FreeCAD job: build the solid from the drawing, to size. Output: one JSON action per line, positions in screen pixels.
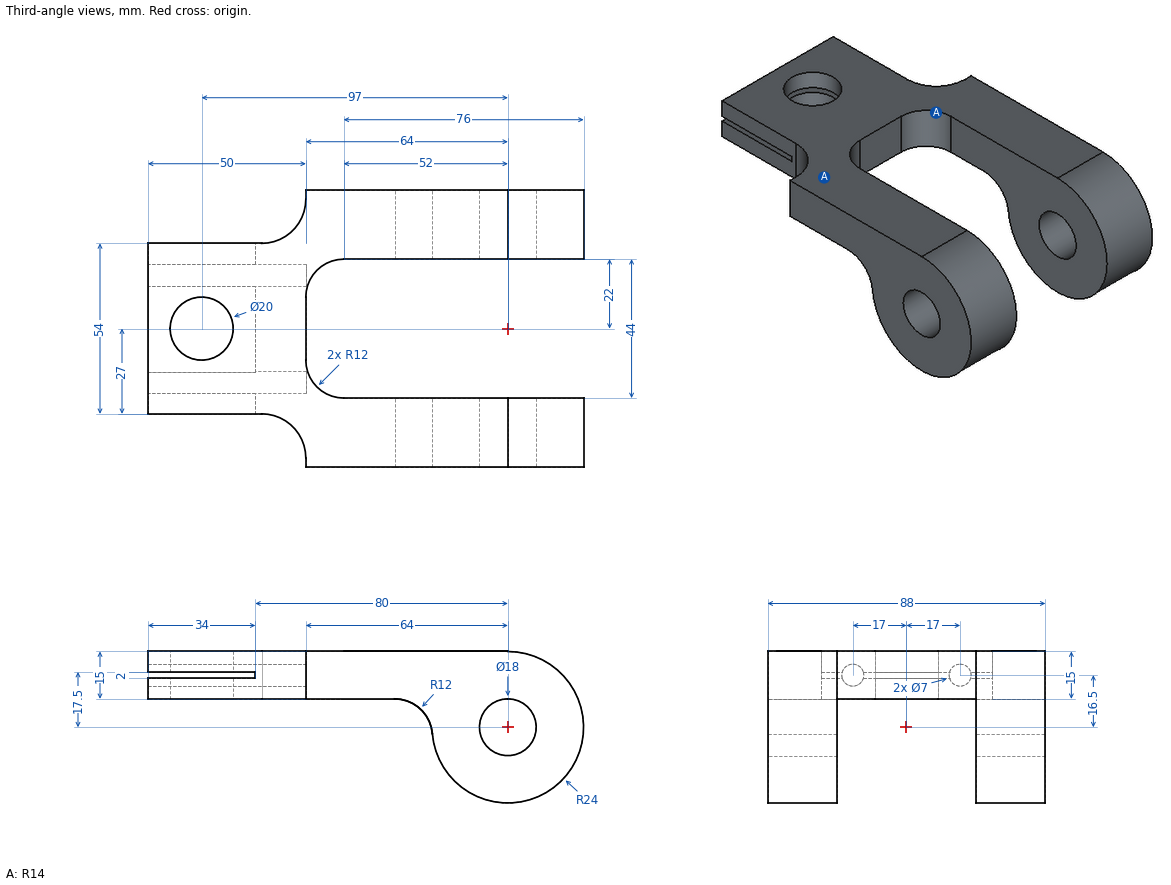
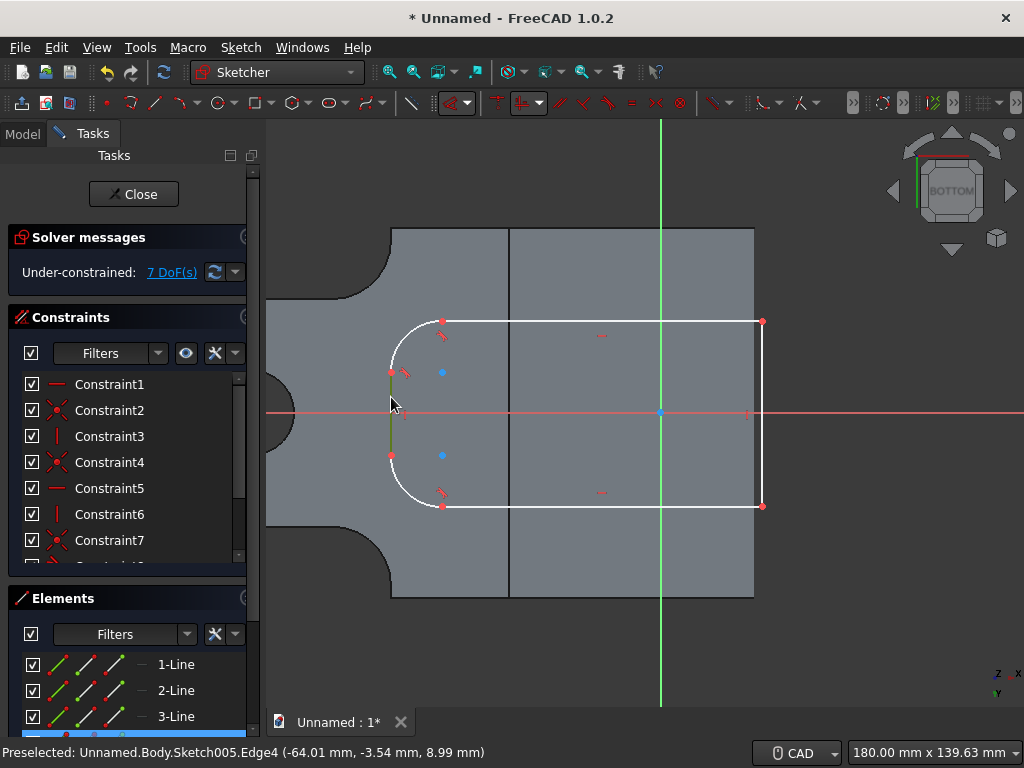
{"action": "left_click", "coordinate": [397, 479]}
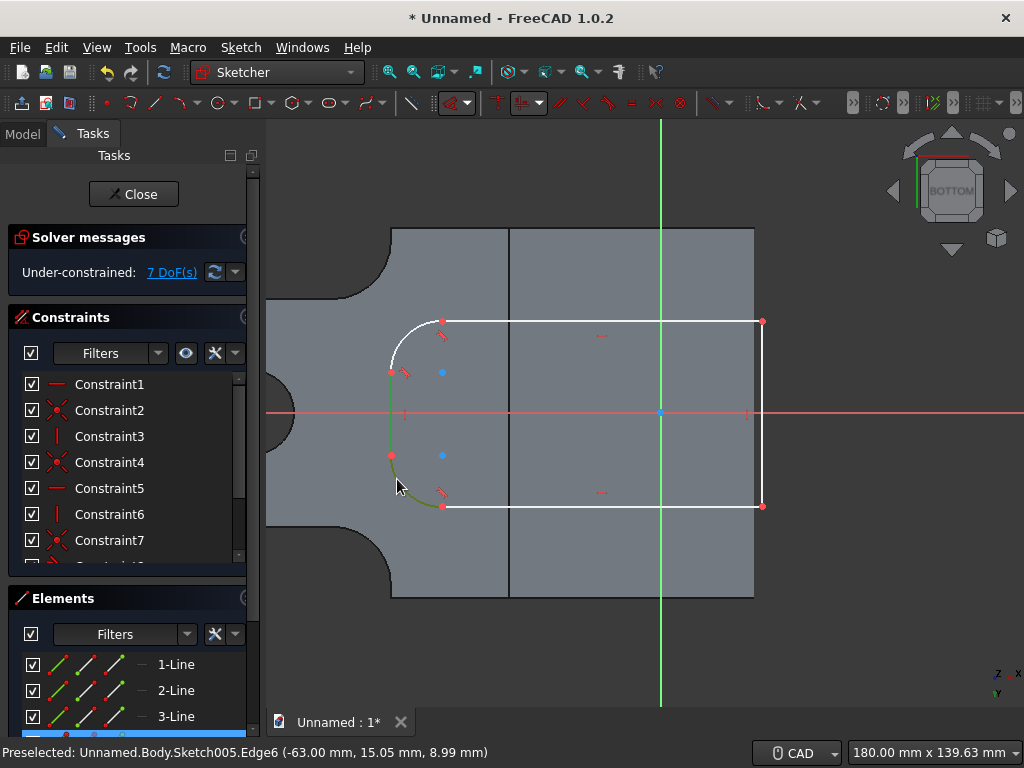
{"action": "left_click", "coordinate": [608, 104]}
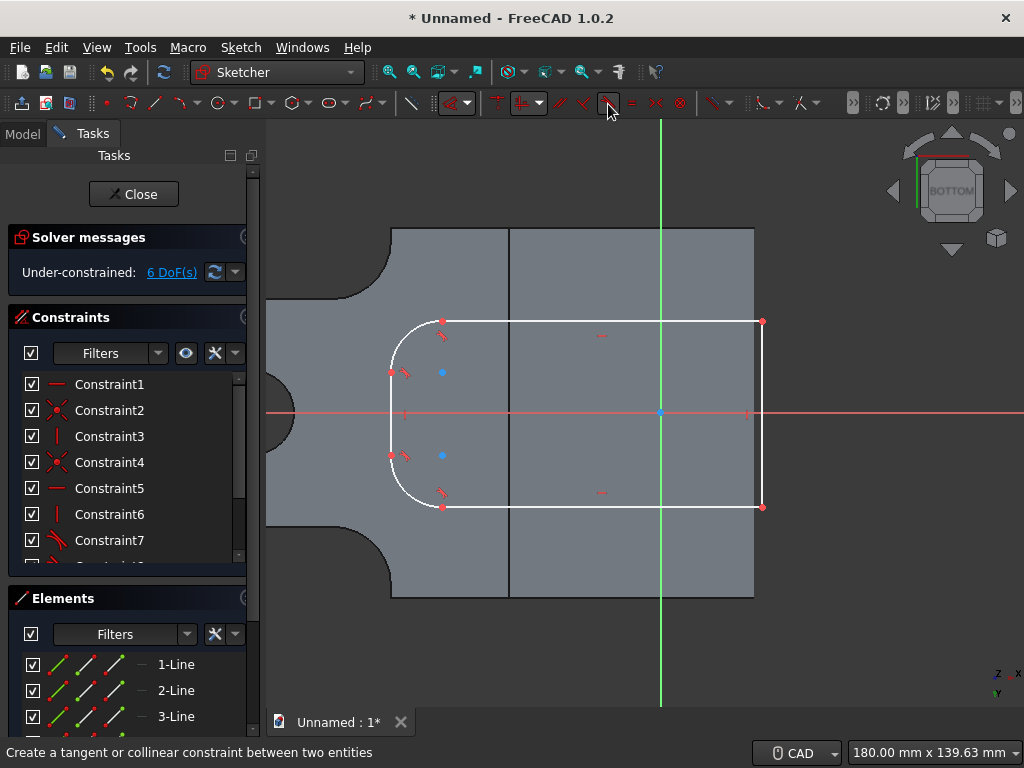
{"action": "left_click", "coordinate": [419, 327]}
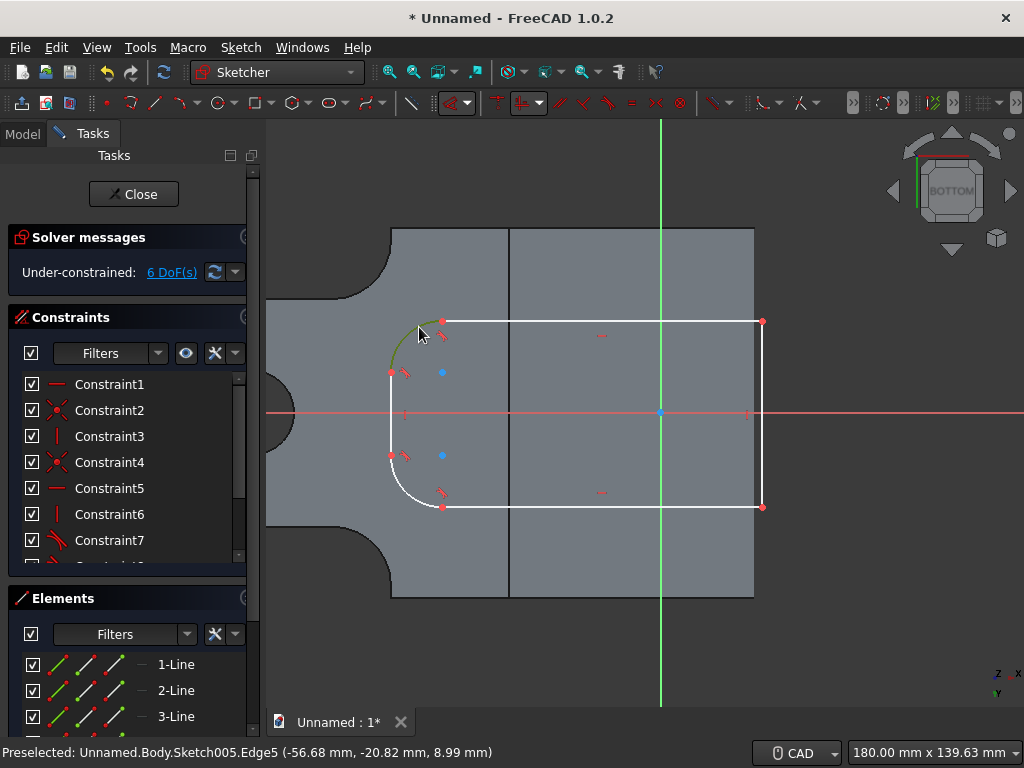
{"action": "left_click", "coordinate": [397, 479]}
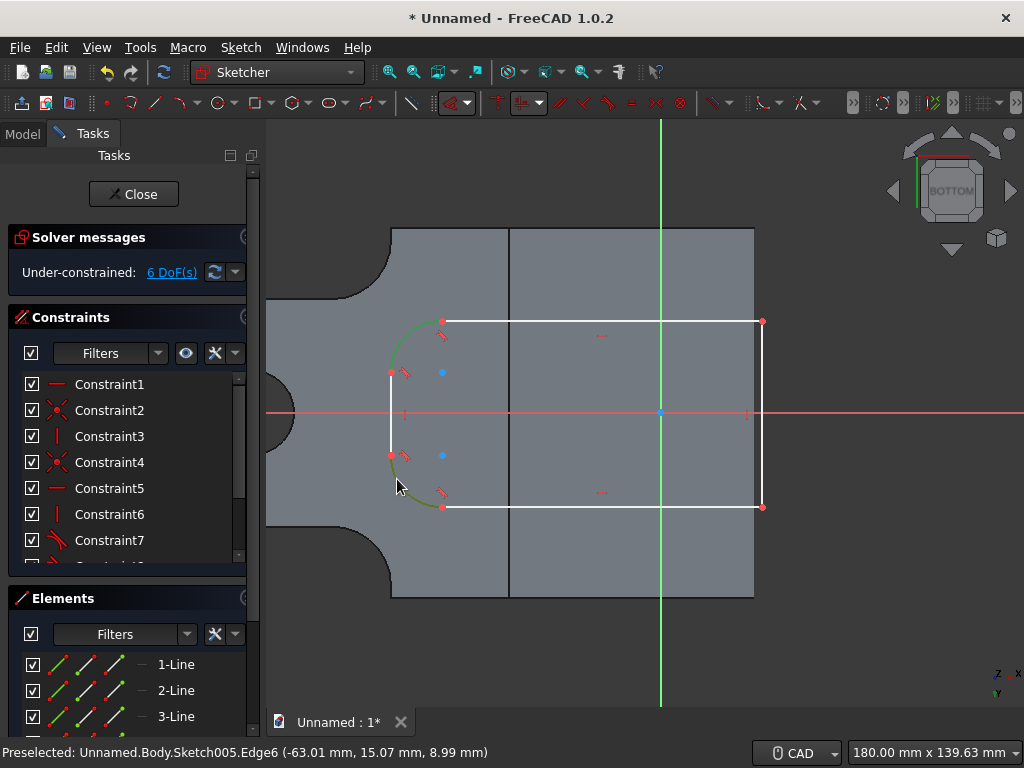
{"action": "left_click", "coordinate": [632, 104]}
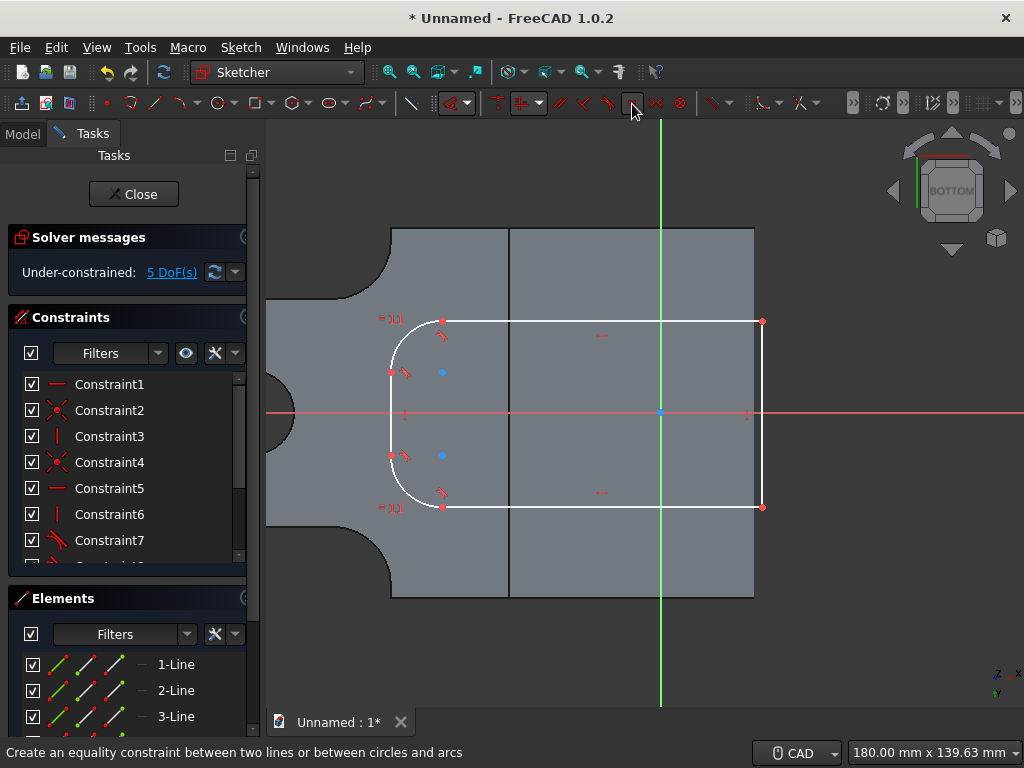
{"action": "left_click", "coordinate": [419, 327]}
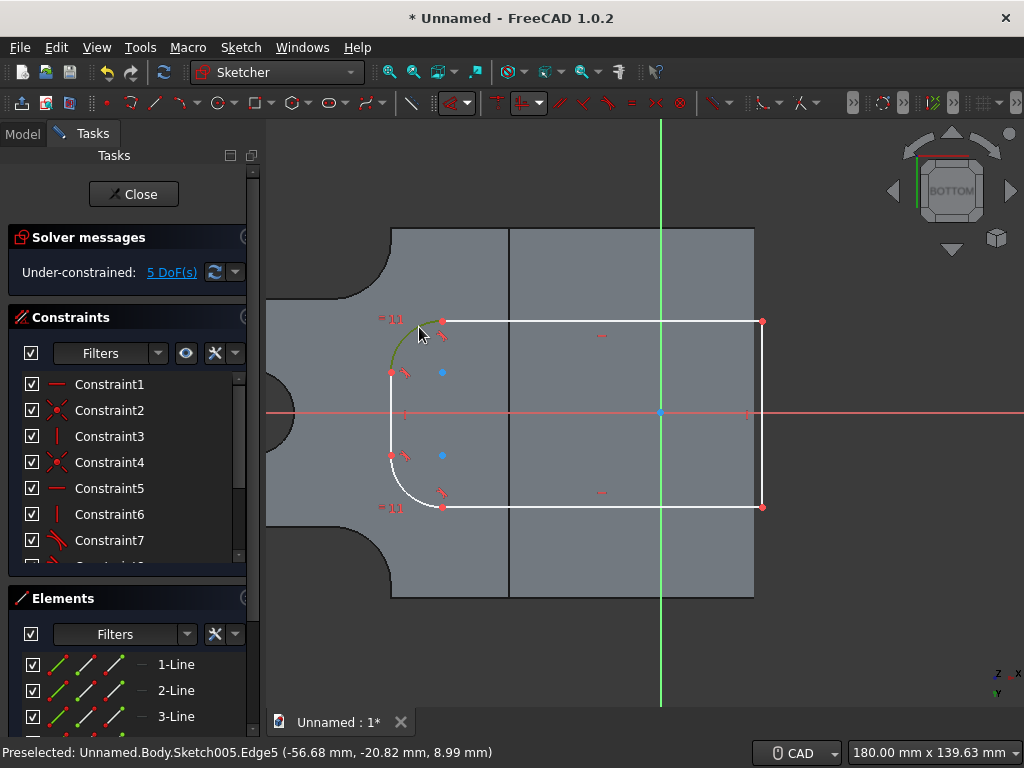
{"action": "left_click", "coordinate": [470, 104]}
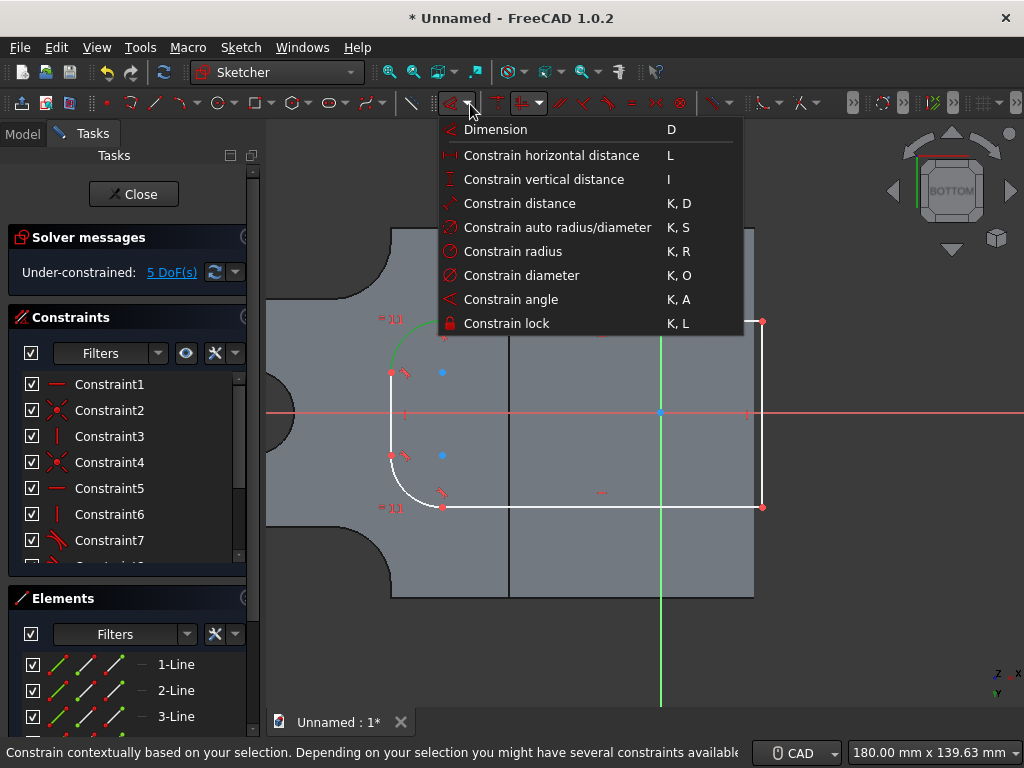
{"action": "left_click", "coordinate": [591, 251]}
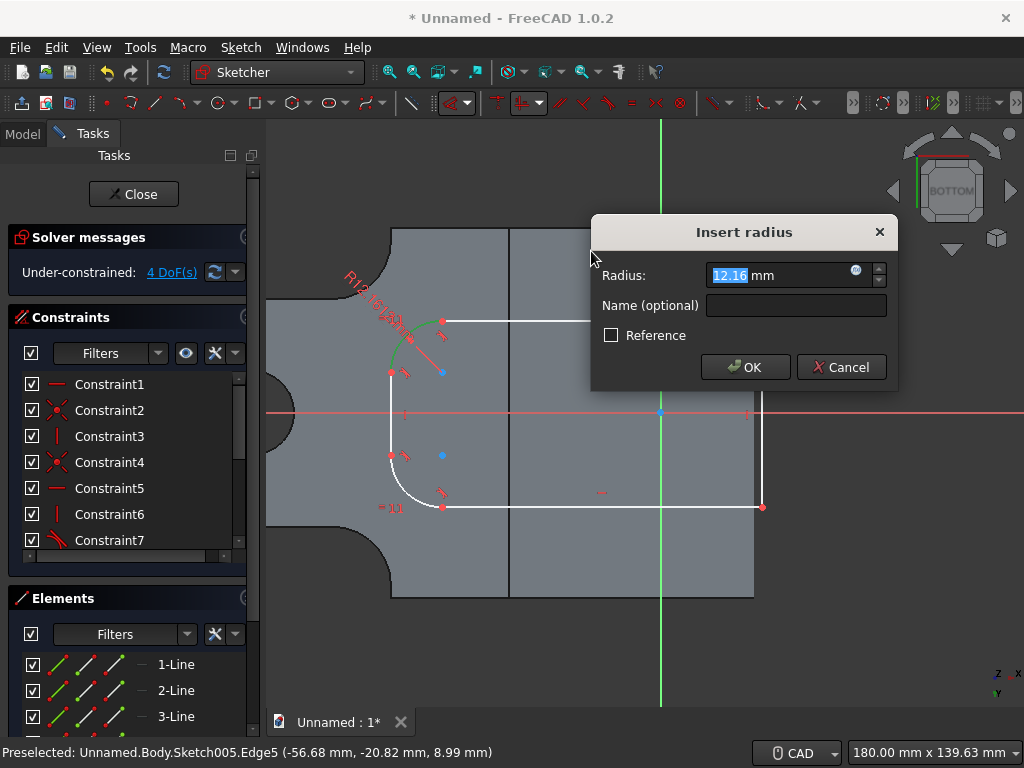
{"action": "type", "text": "12"}
{"action": "key", "text": "Return"}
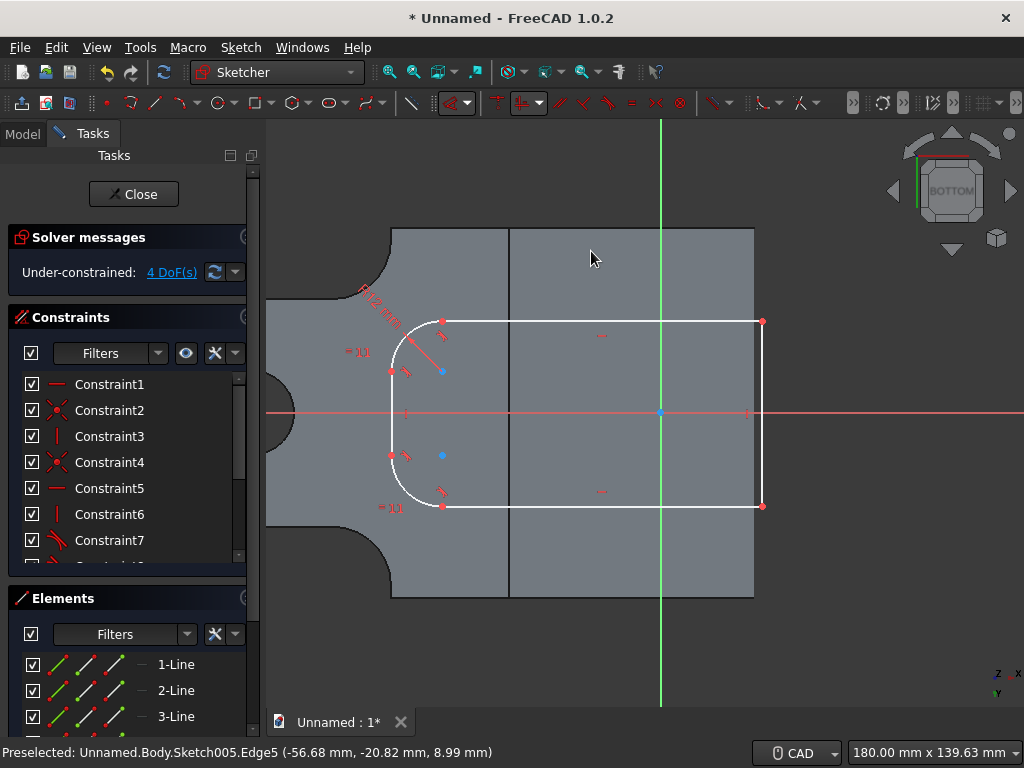
{"action": "left_click", "coordinate": [538, 507]}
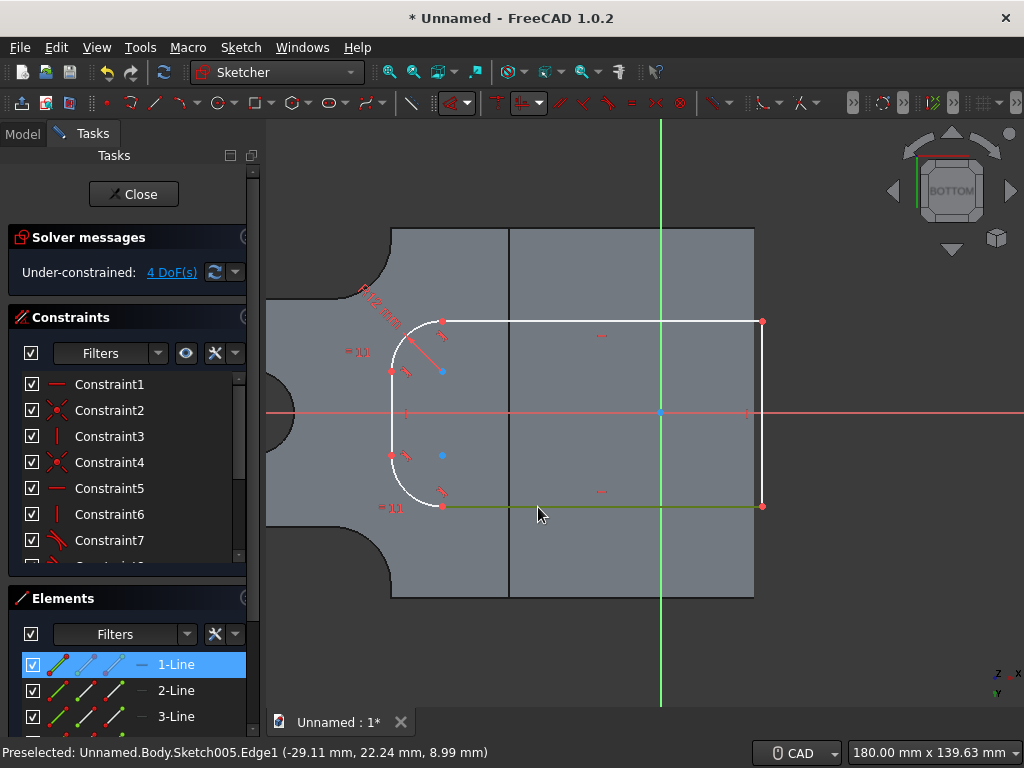
{"action": "left_click", "coordinate": [470, 104]}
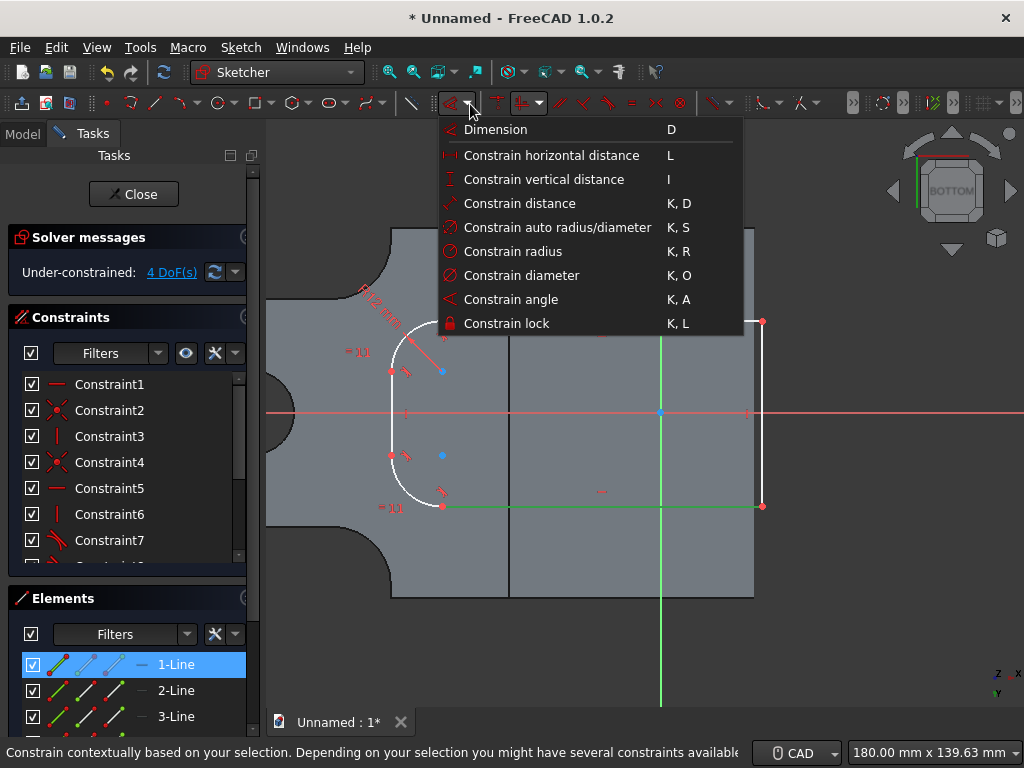
{"action": "left_click", "coordinate": [591, 155]}